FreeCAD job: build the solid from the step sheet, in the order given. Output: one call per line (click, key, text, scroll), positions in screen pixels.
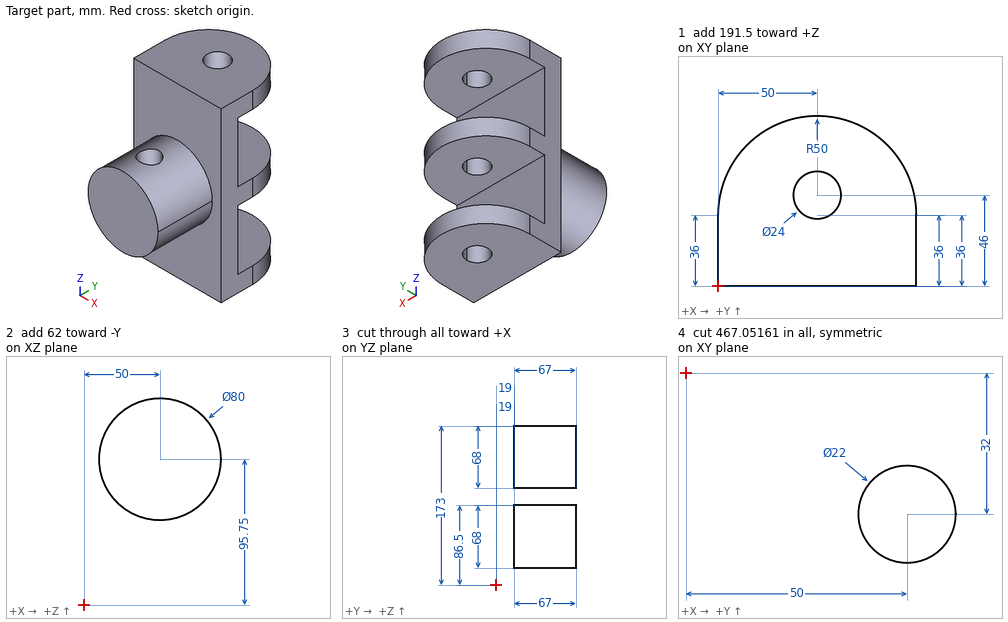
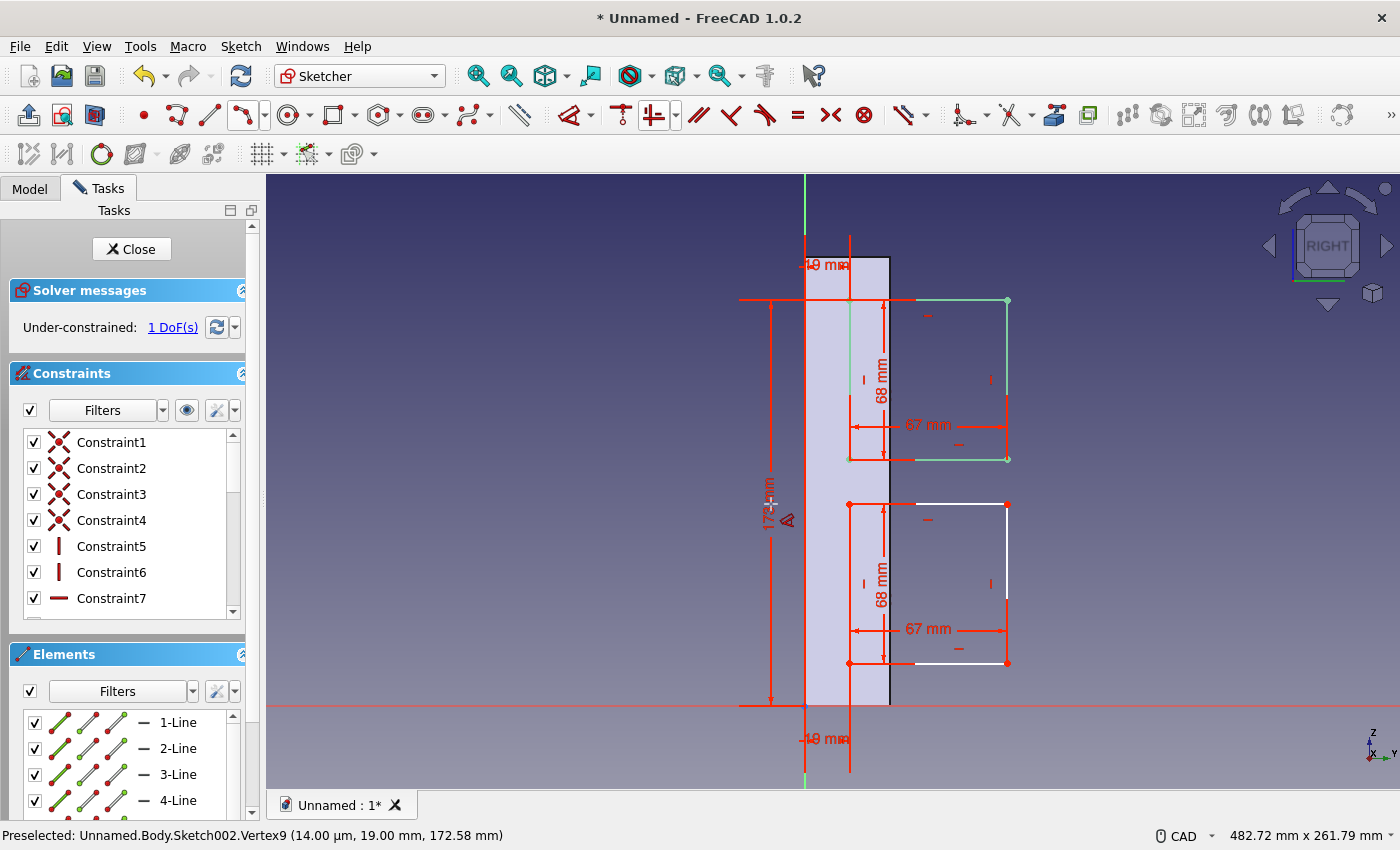
click(850, 504)
click(771, 605)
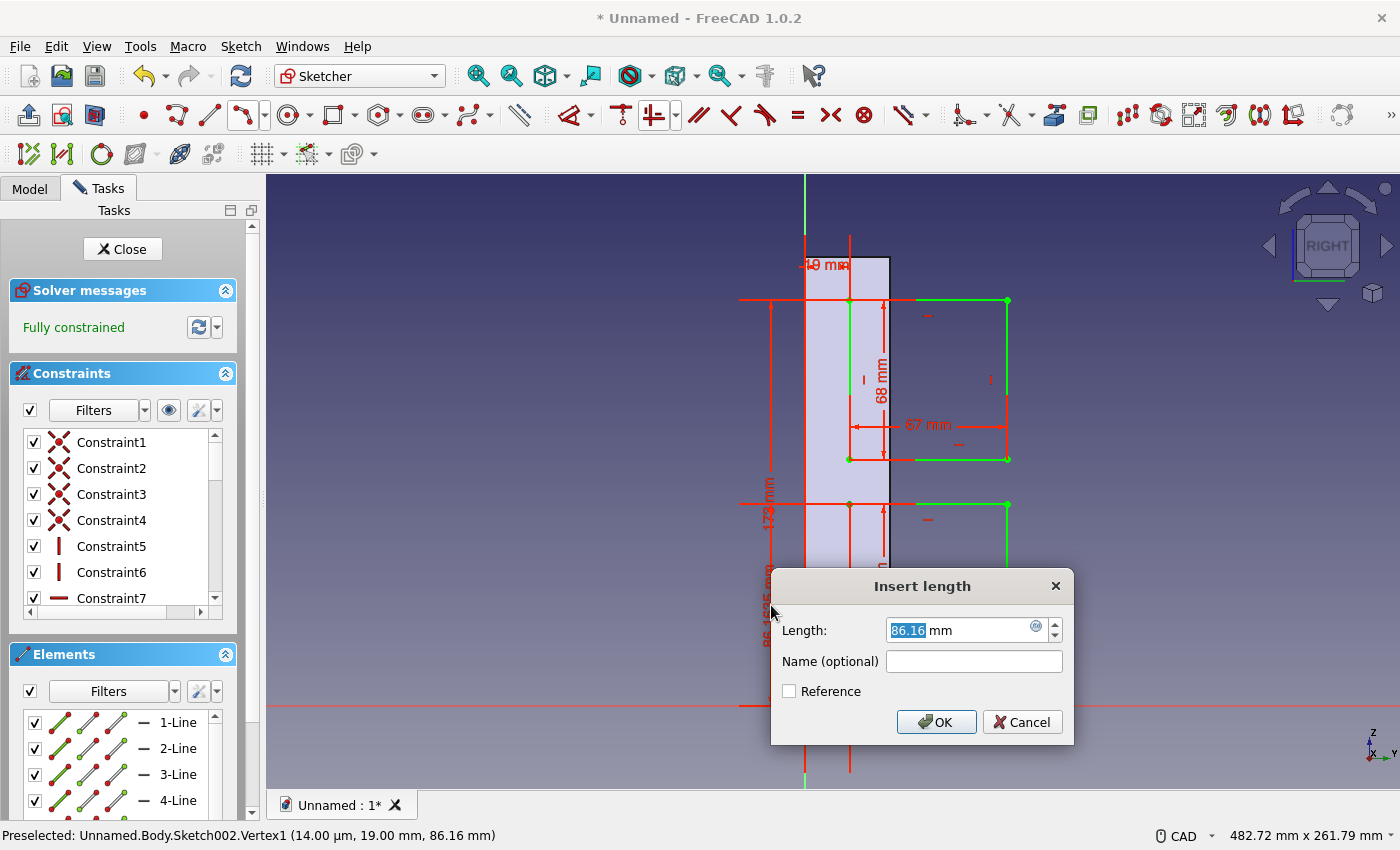
text(86.5)
key(Return)
key(Escape)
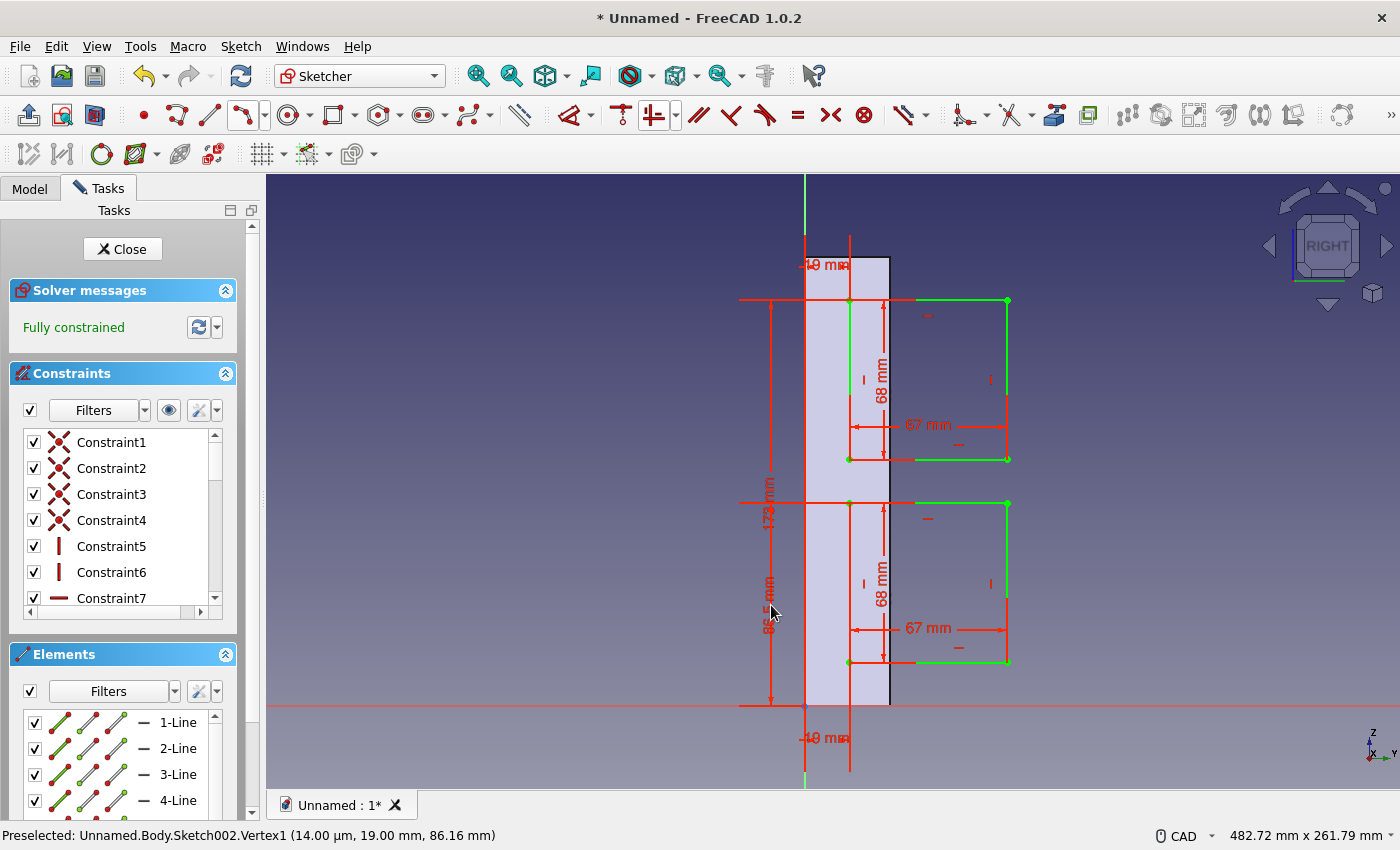
click(123, 249)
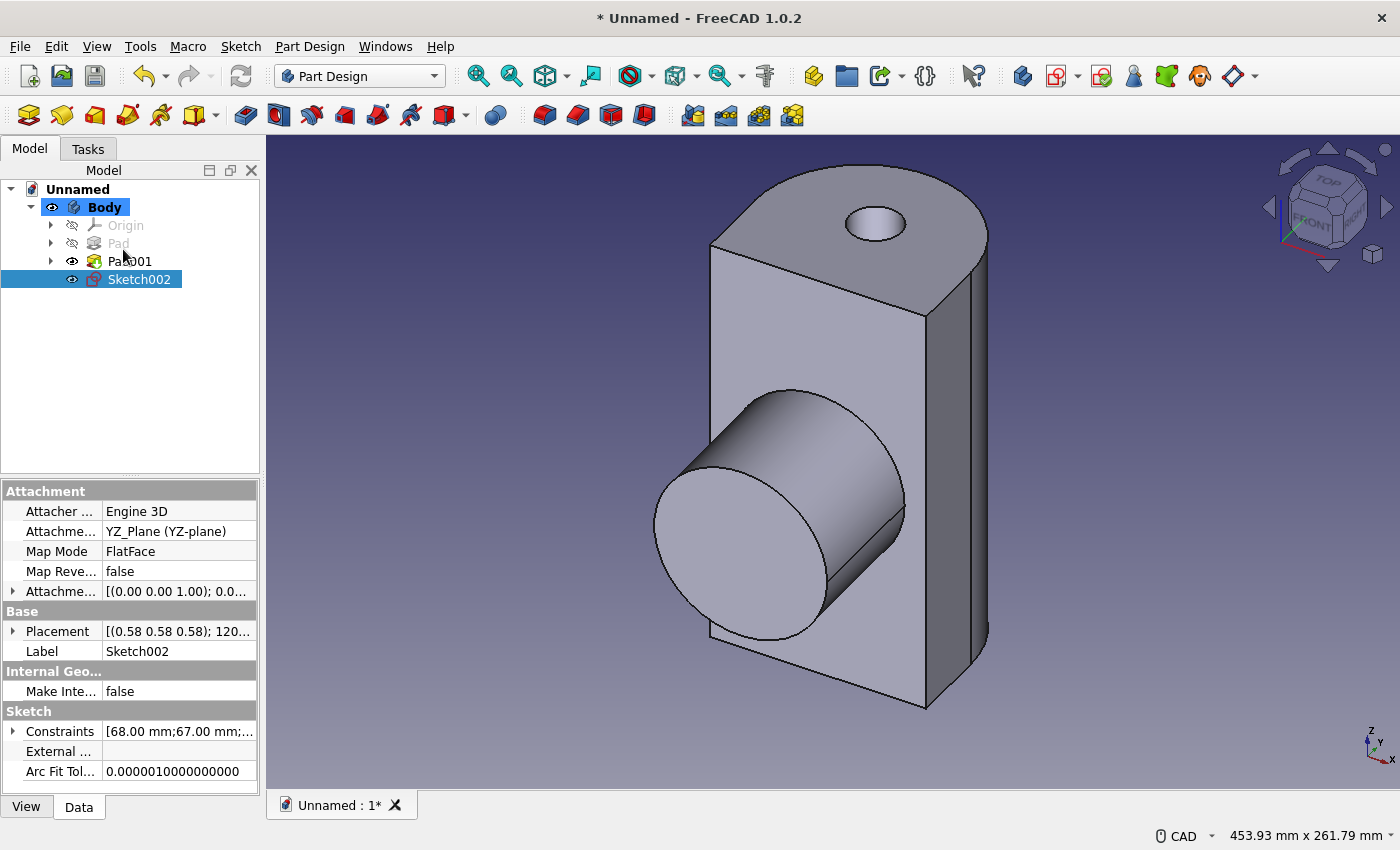
click(246, 116)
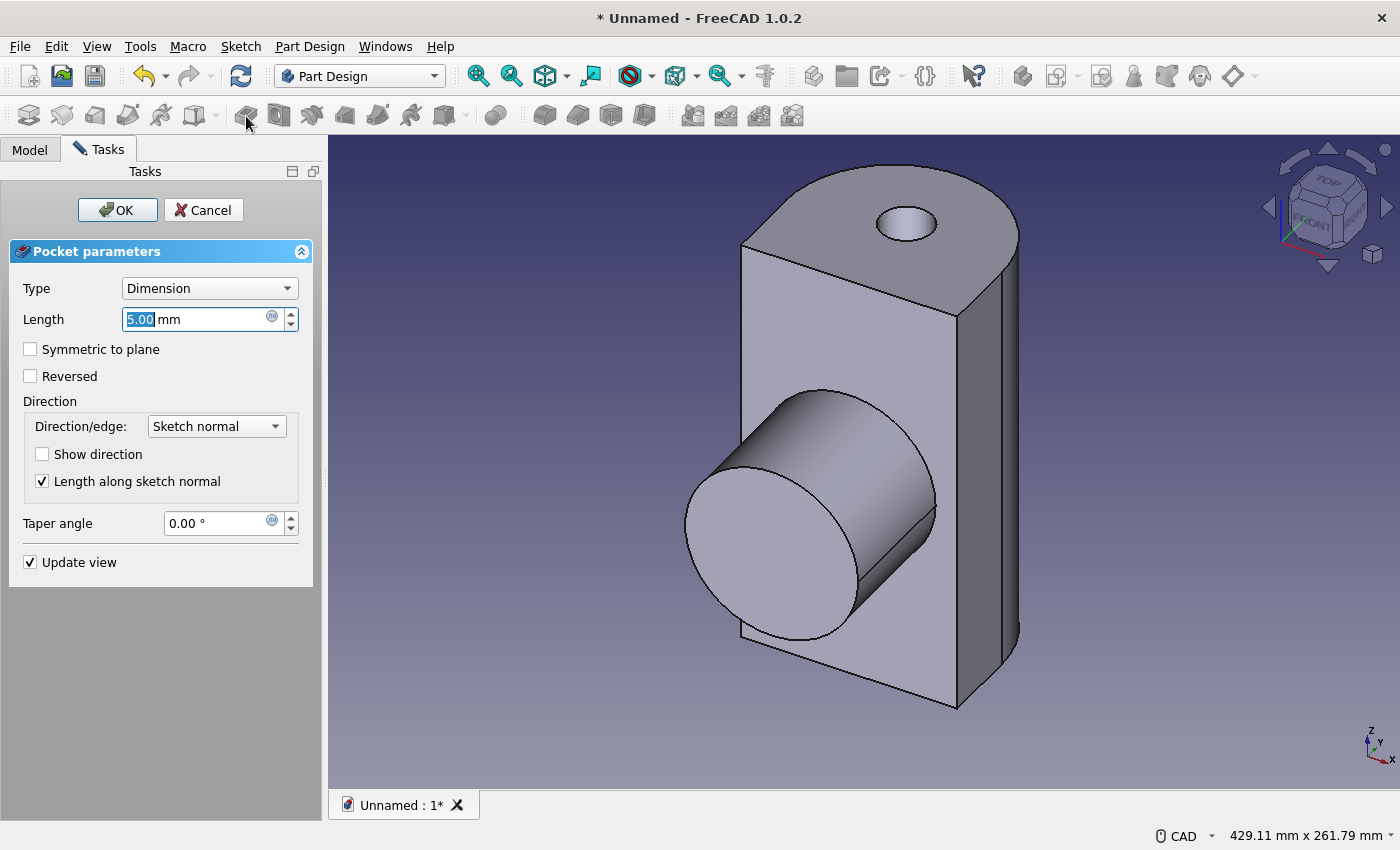
click(210, 288)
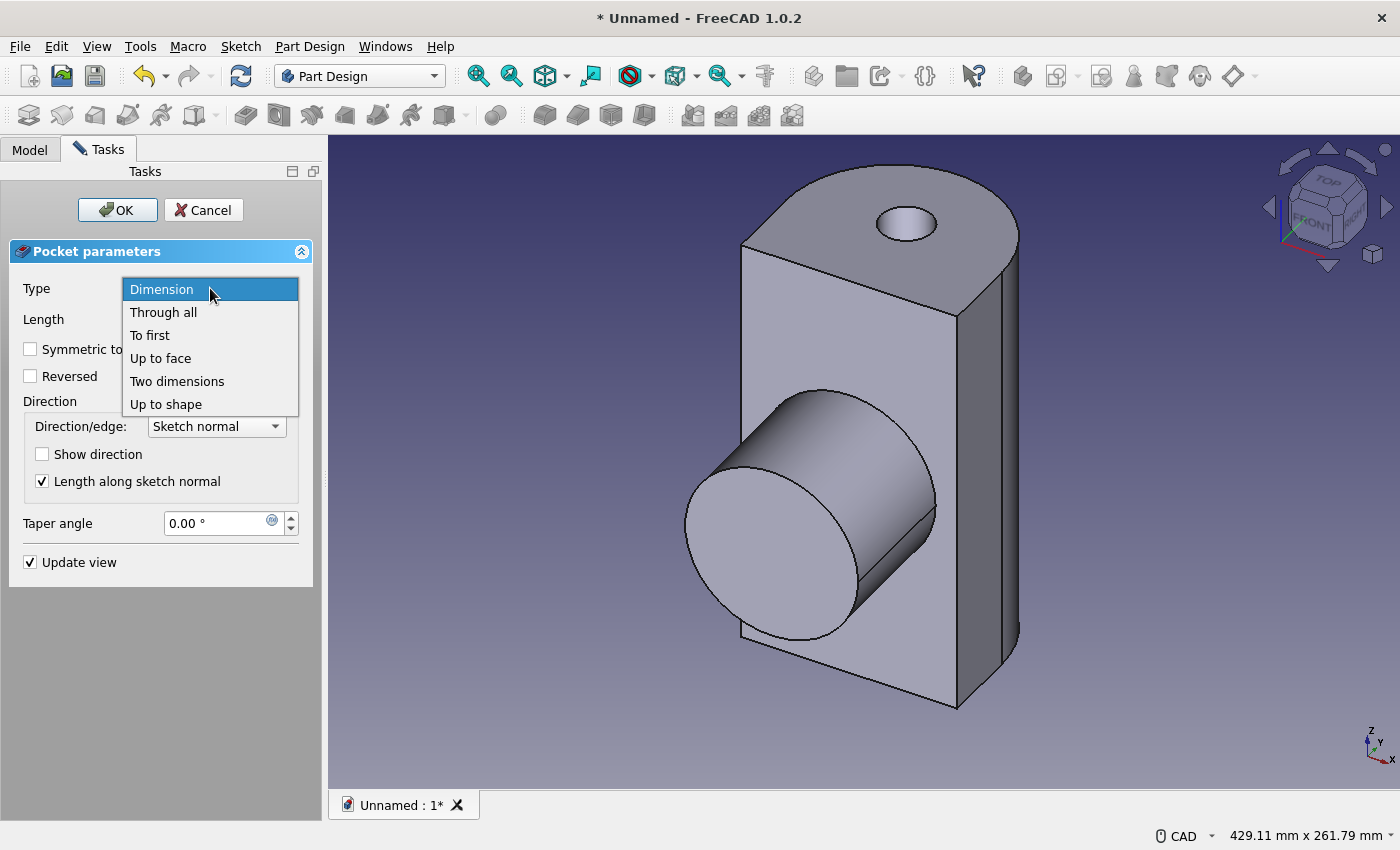
click(208, 312)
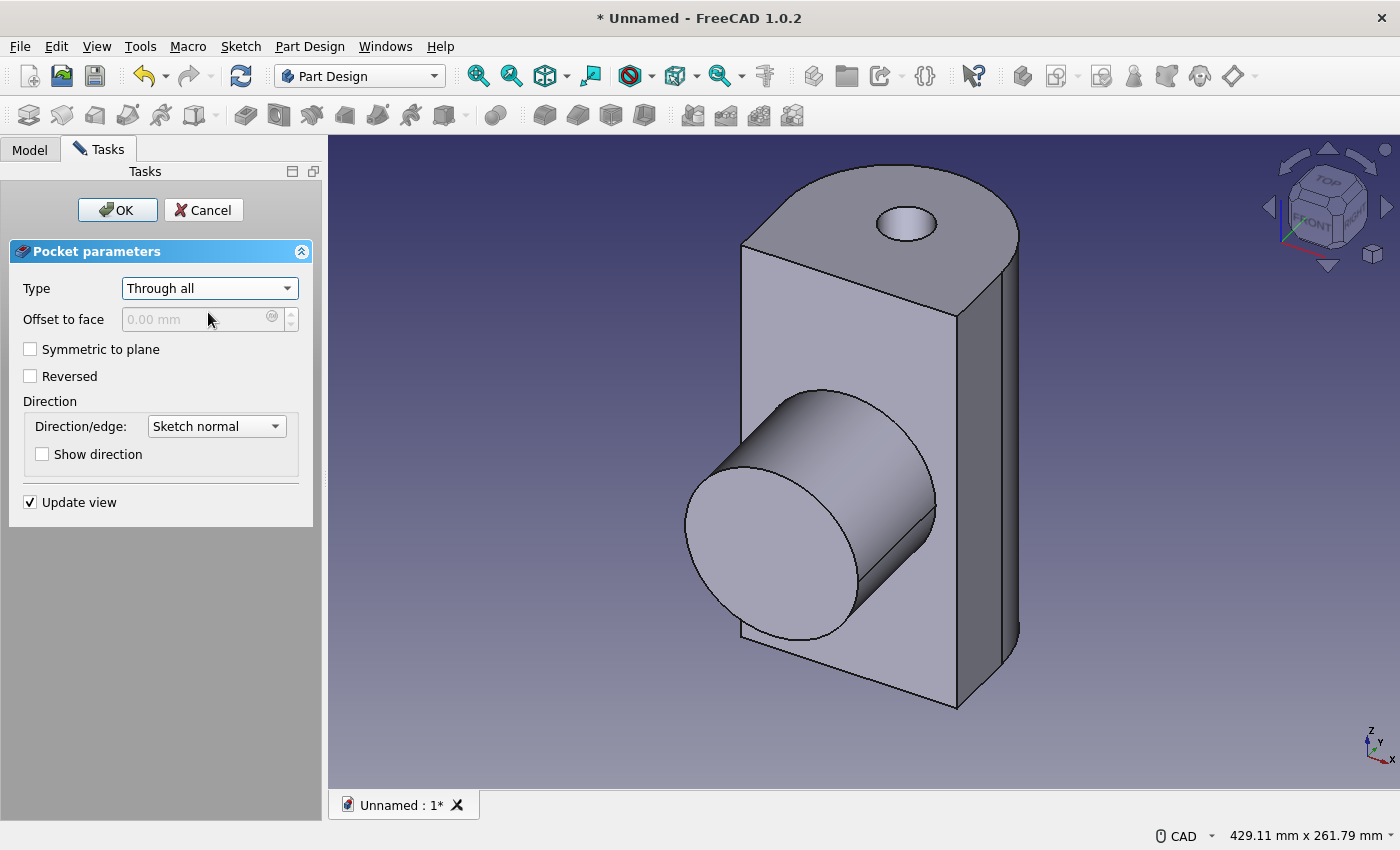
click(31, 376)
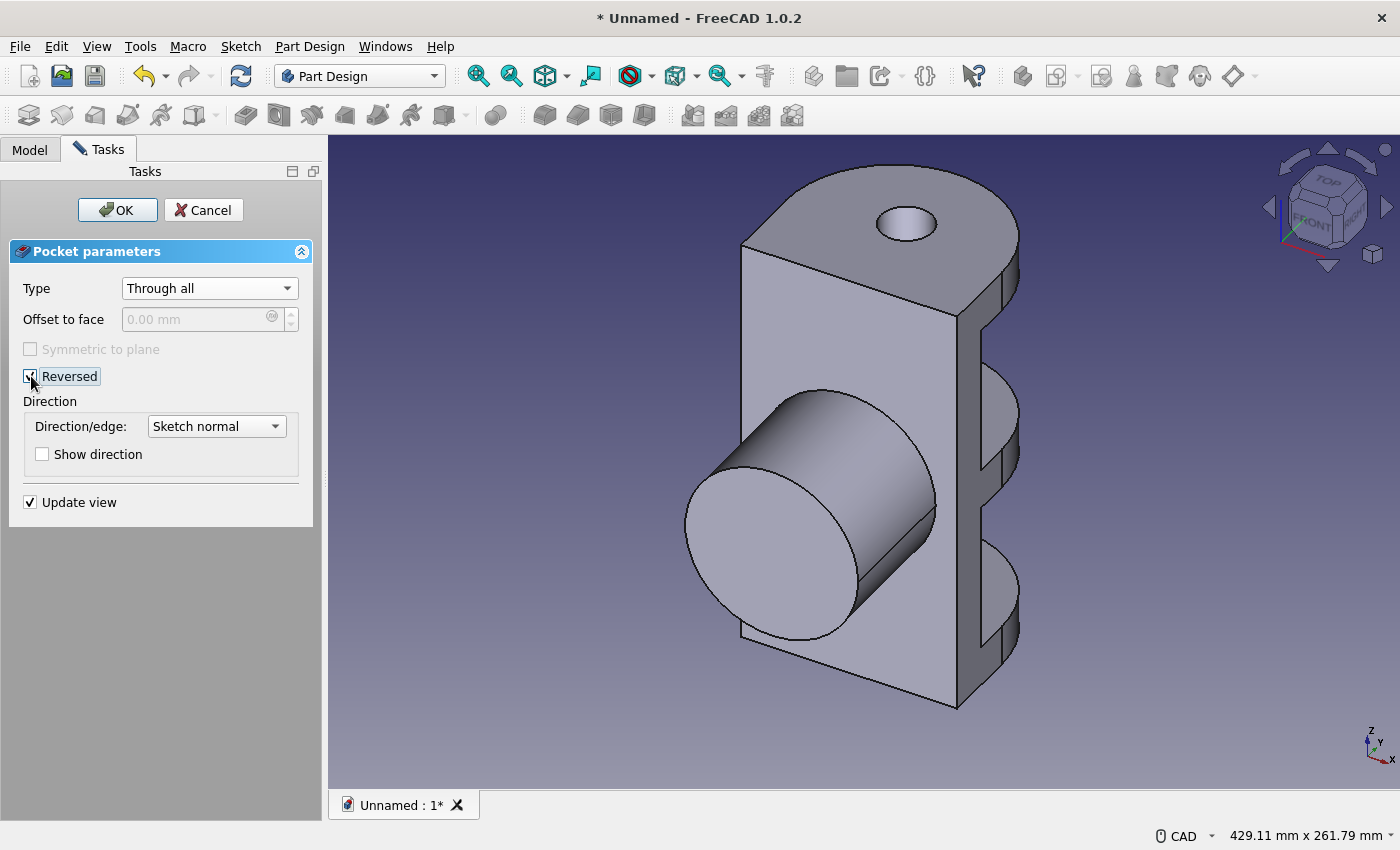
click(118, 210)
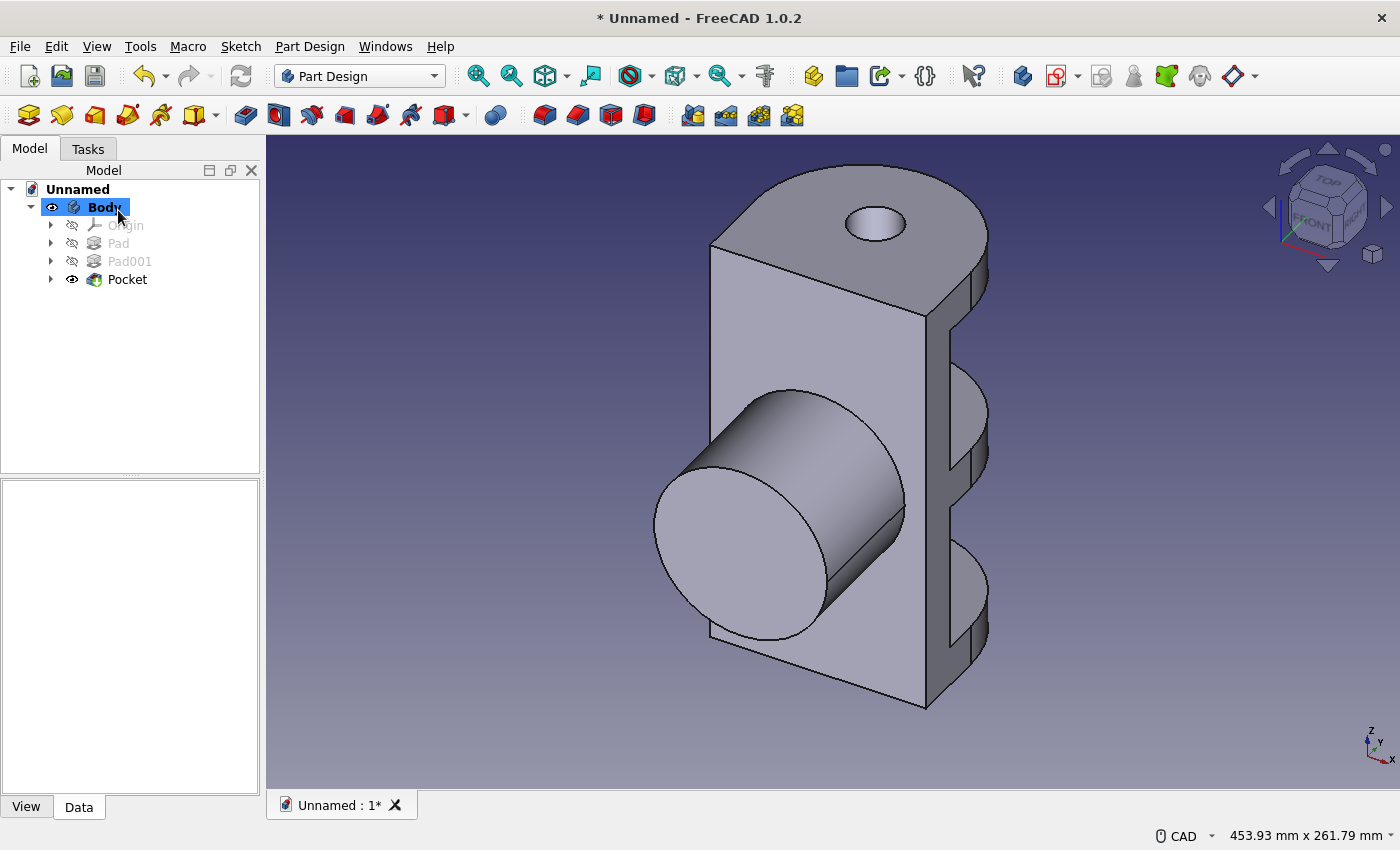
click(1056, 76)